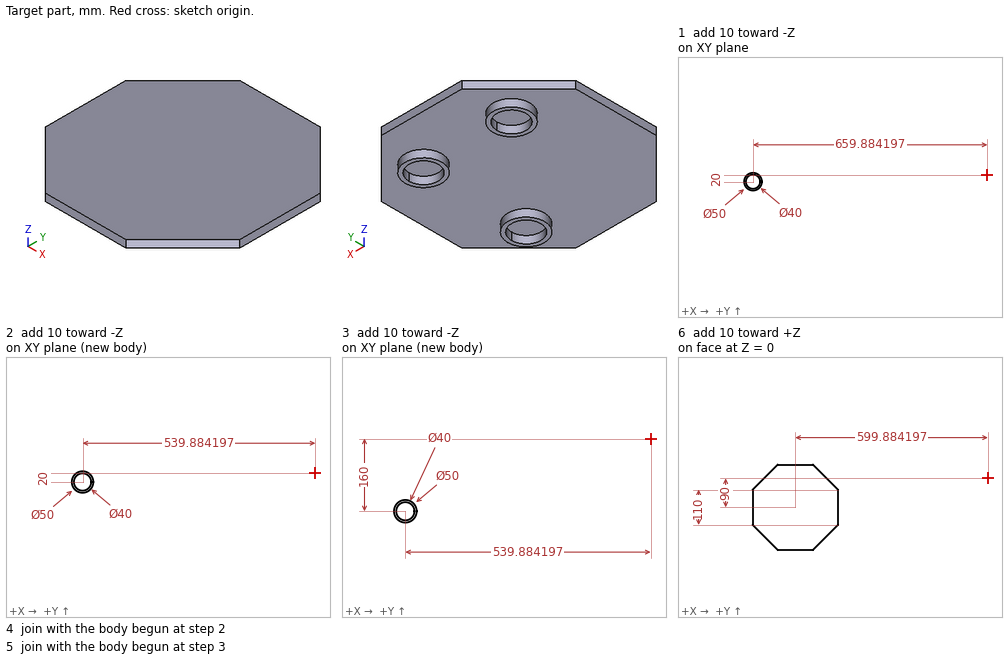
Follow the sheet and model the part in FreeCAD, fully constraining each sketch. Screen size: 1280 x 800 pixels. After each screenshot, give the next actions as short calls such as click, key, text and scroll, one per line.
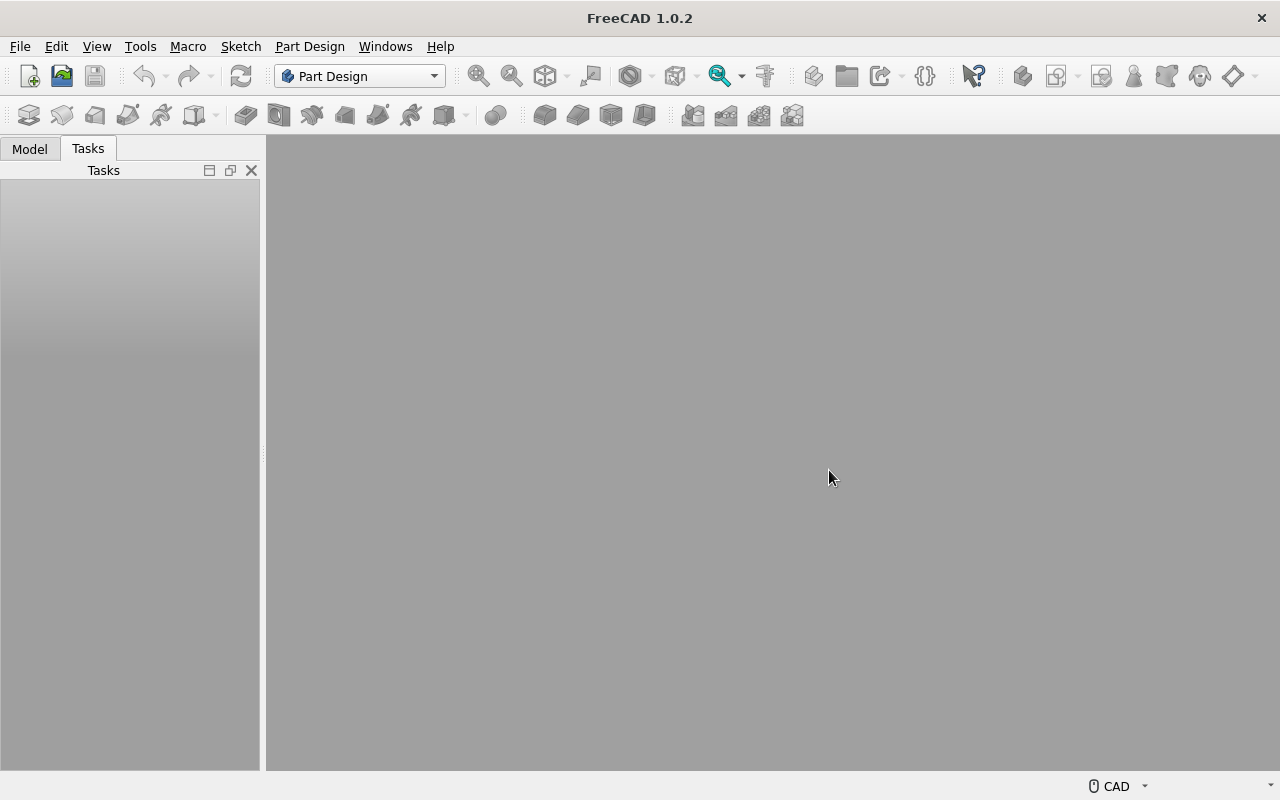
key(ctrl+n)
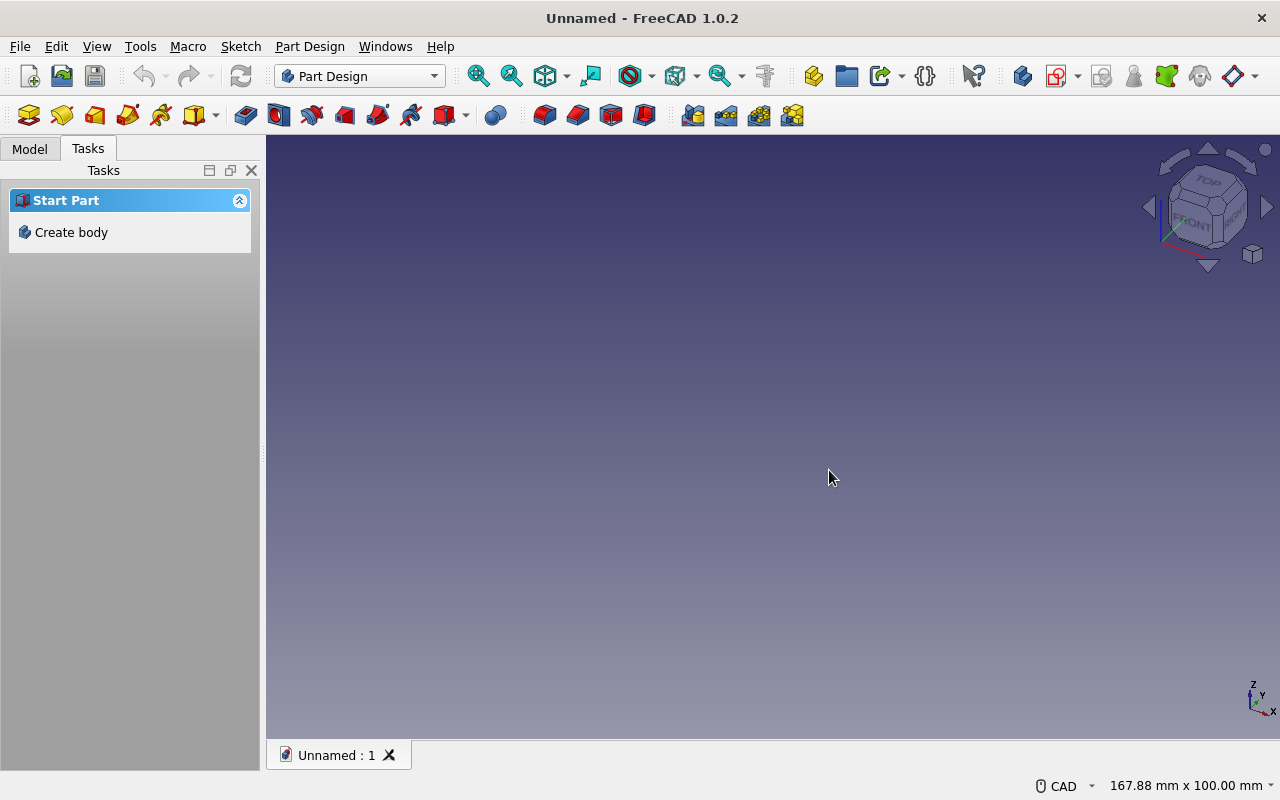
click(1056, 76)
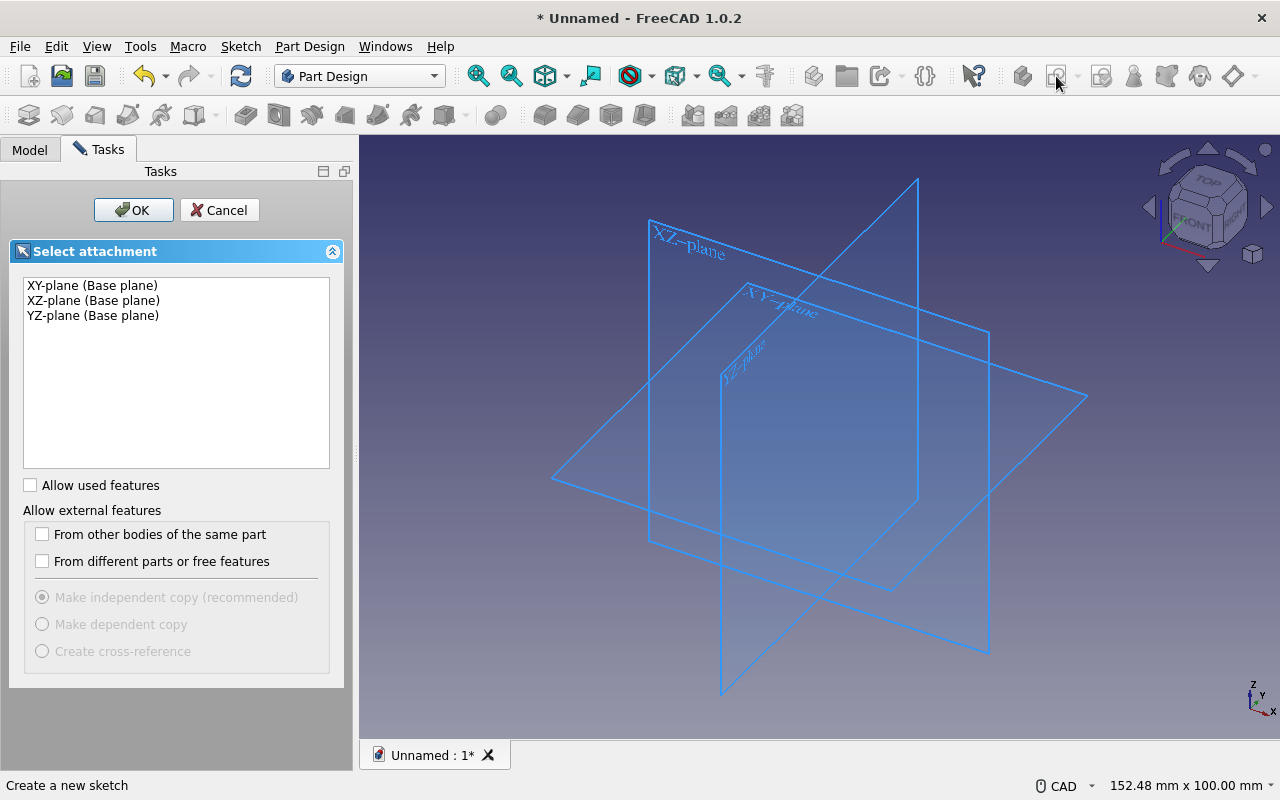
click(84, 286)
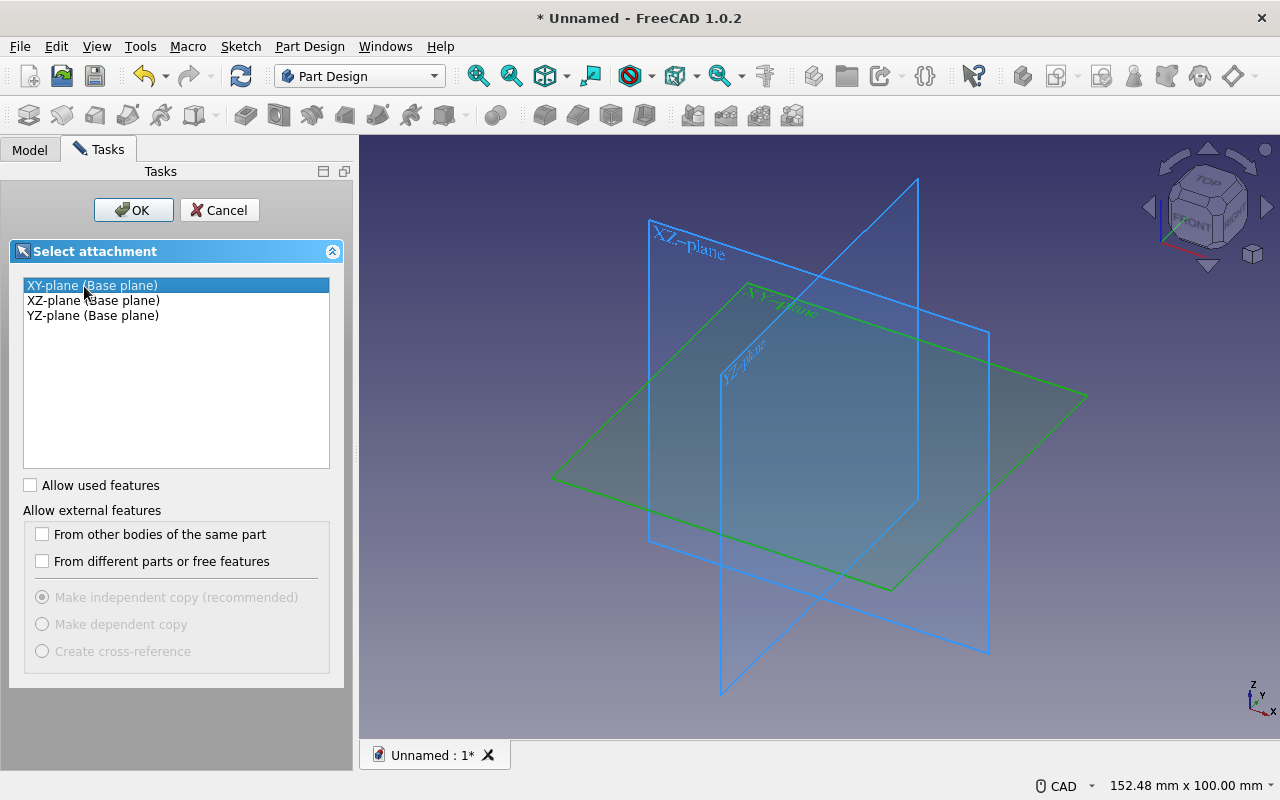
click(134, 210)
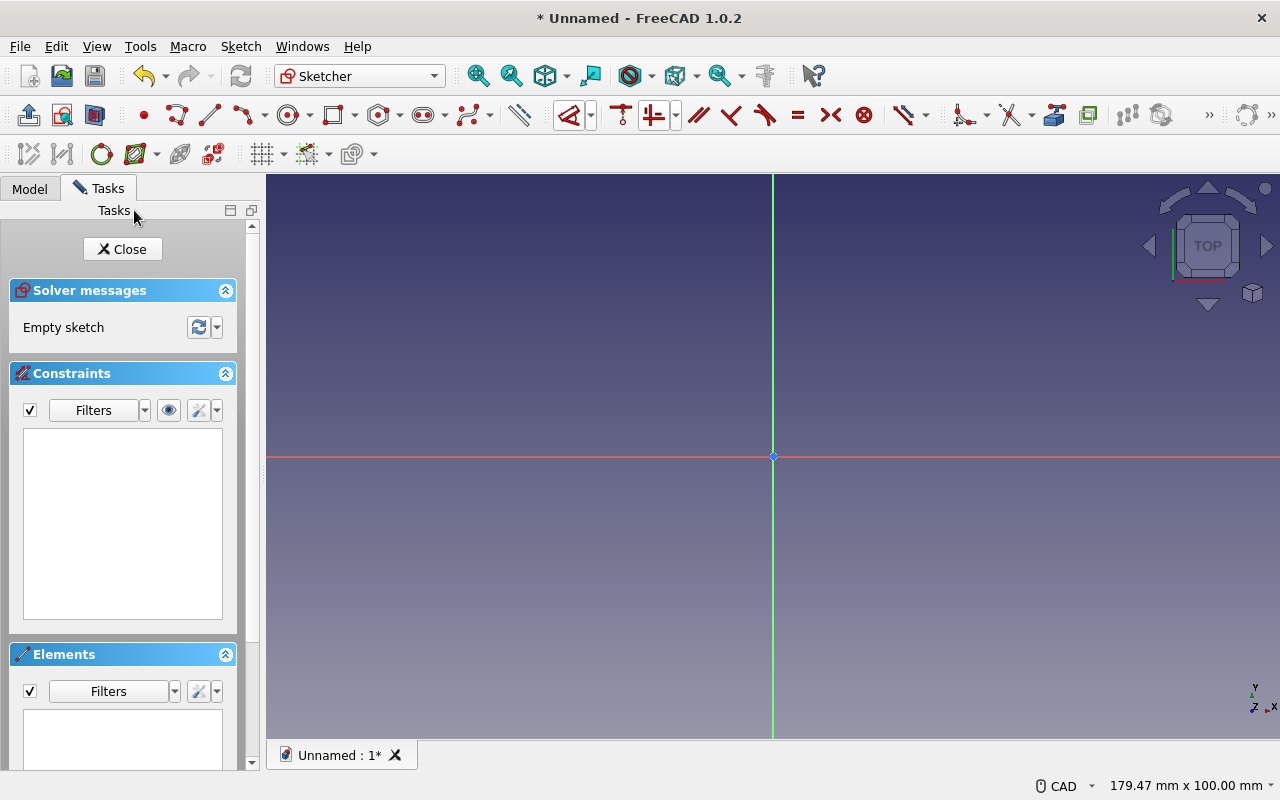
scroll(704, 456, down, 5)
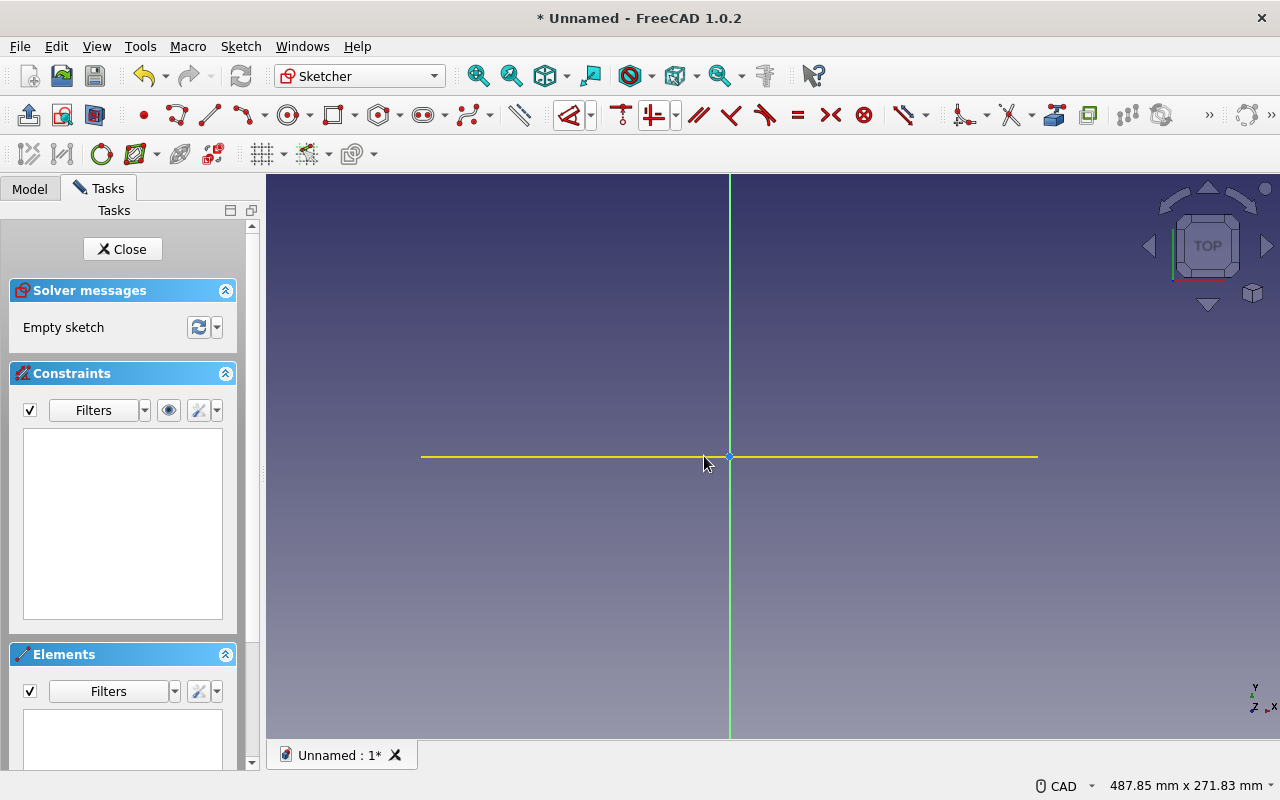
scroll(704, 456, down, 5)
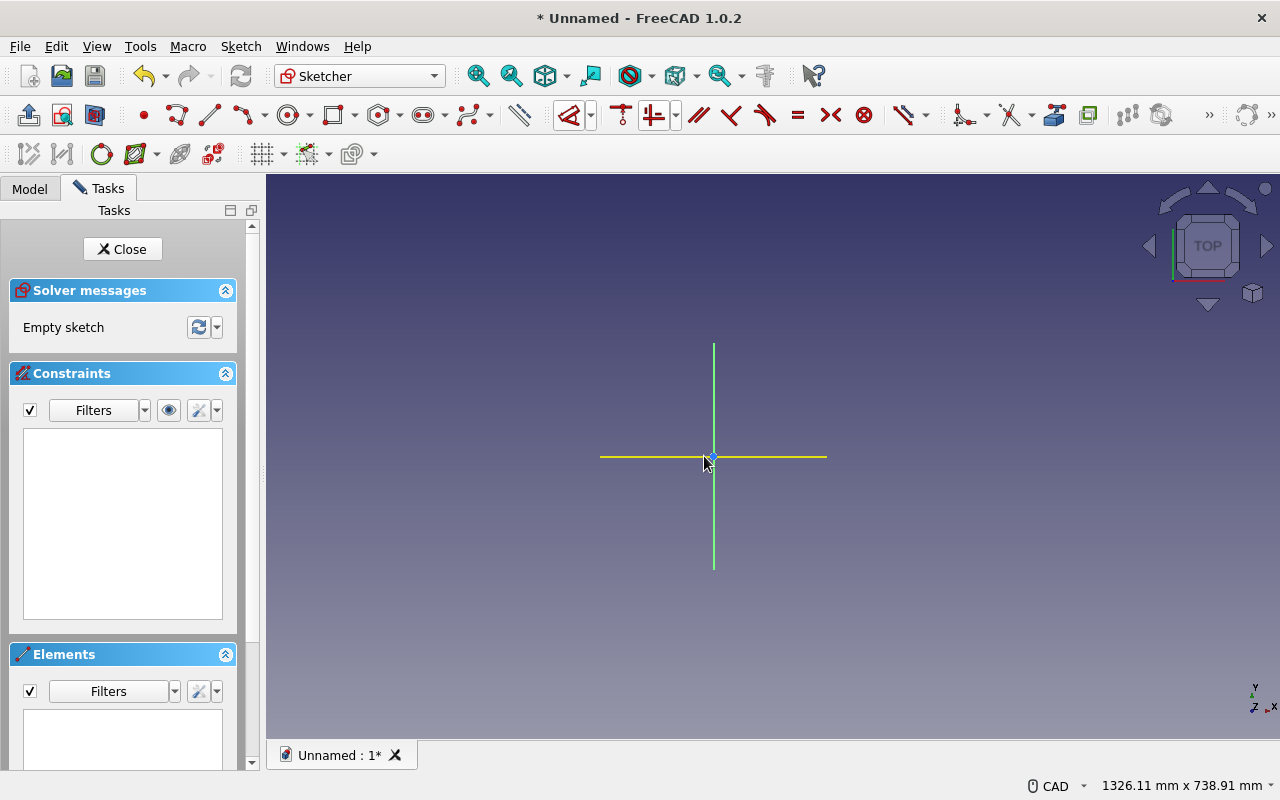
scroll(704, 456, down, 5)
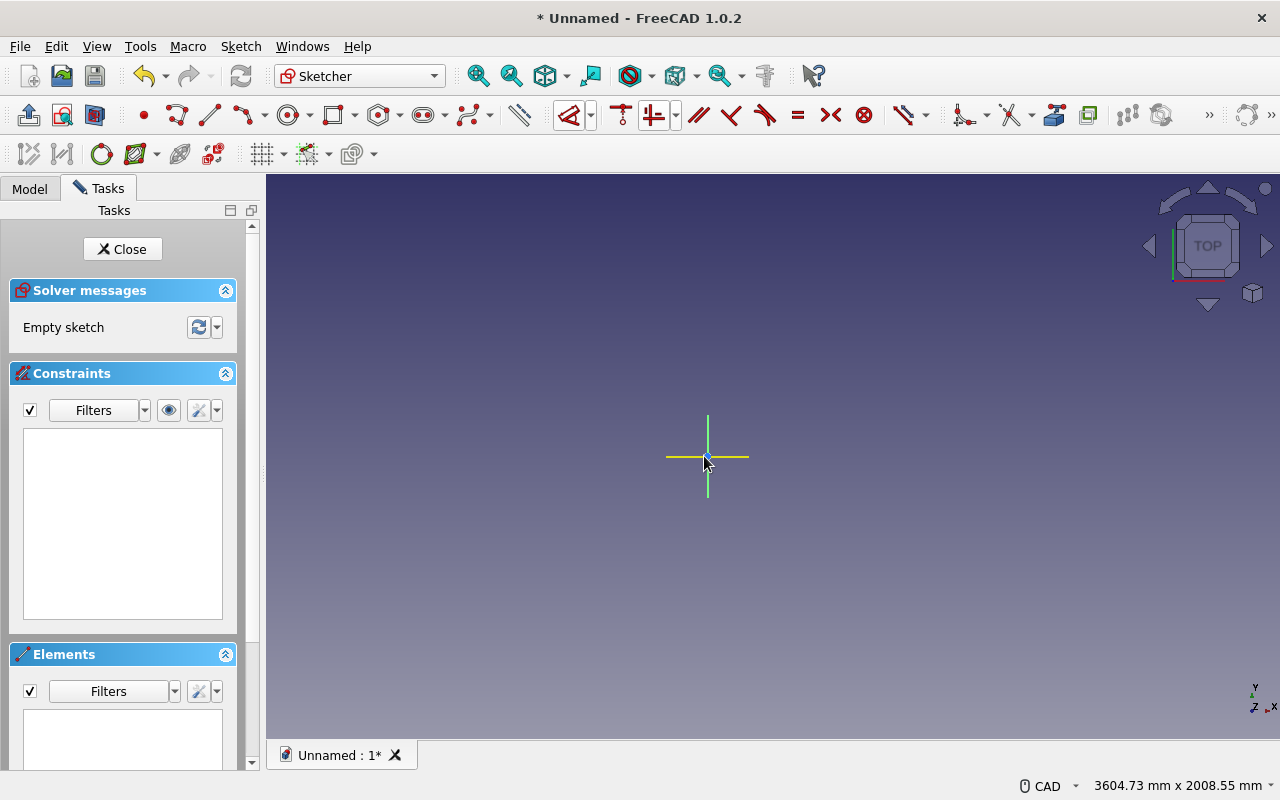
scroll(513, 462, up, 15)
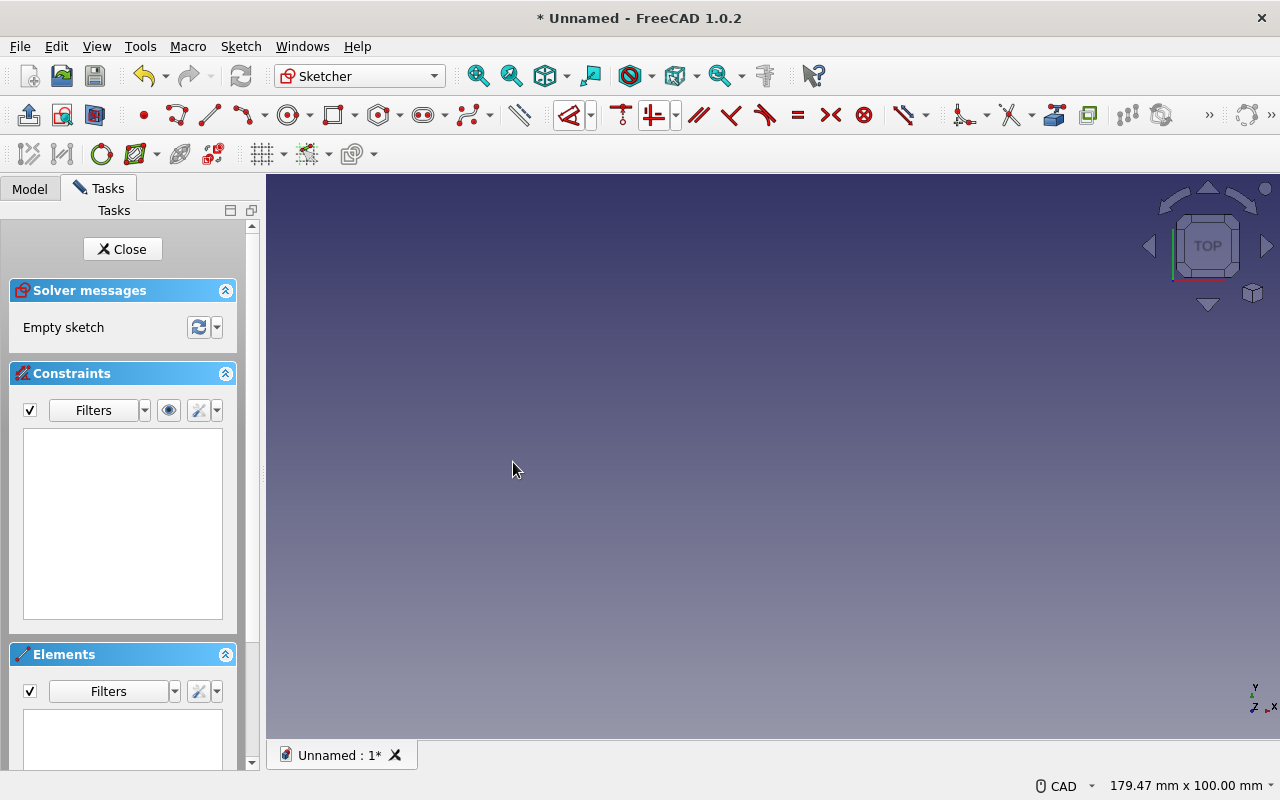
key(g)
key(c)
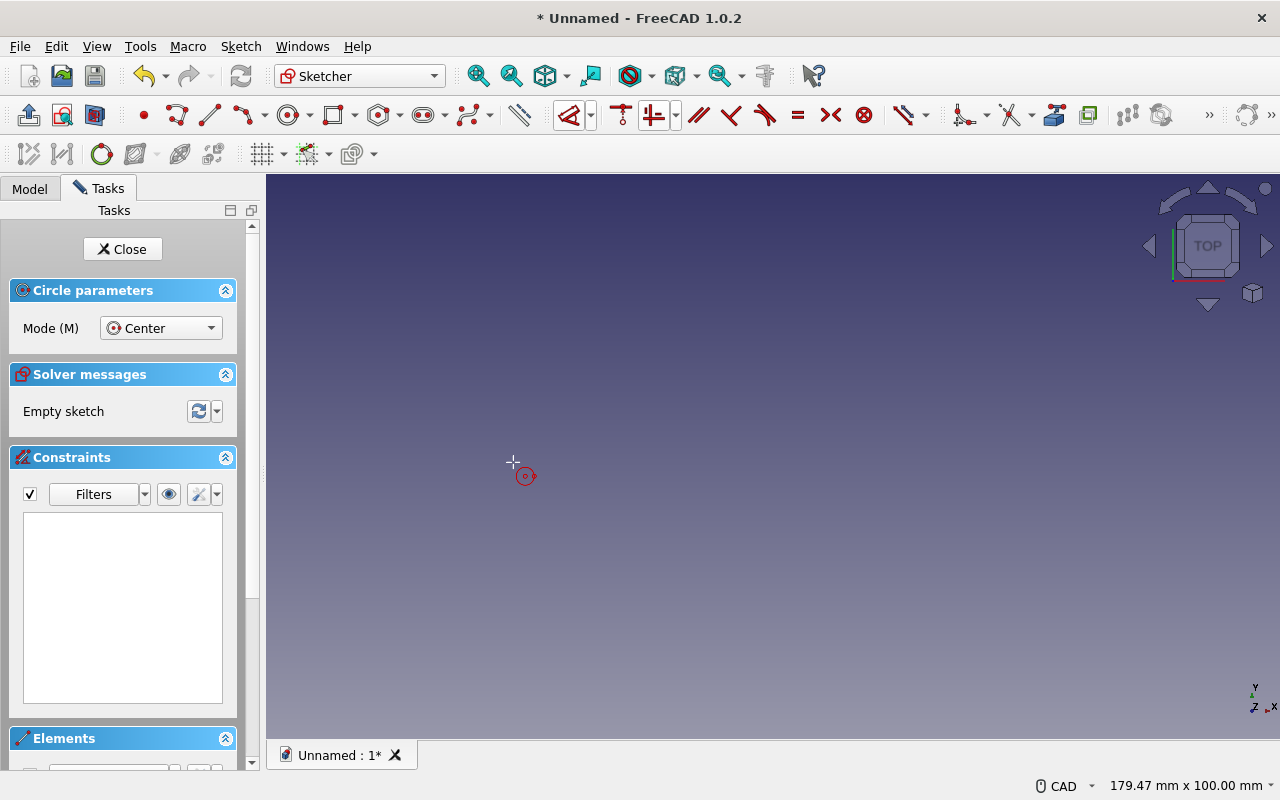
click(694, 455)
move(793, 555)